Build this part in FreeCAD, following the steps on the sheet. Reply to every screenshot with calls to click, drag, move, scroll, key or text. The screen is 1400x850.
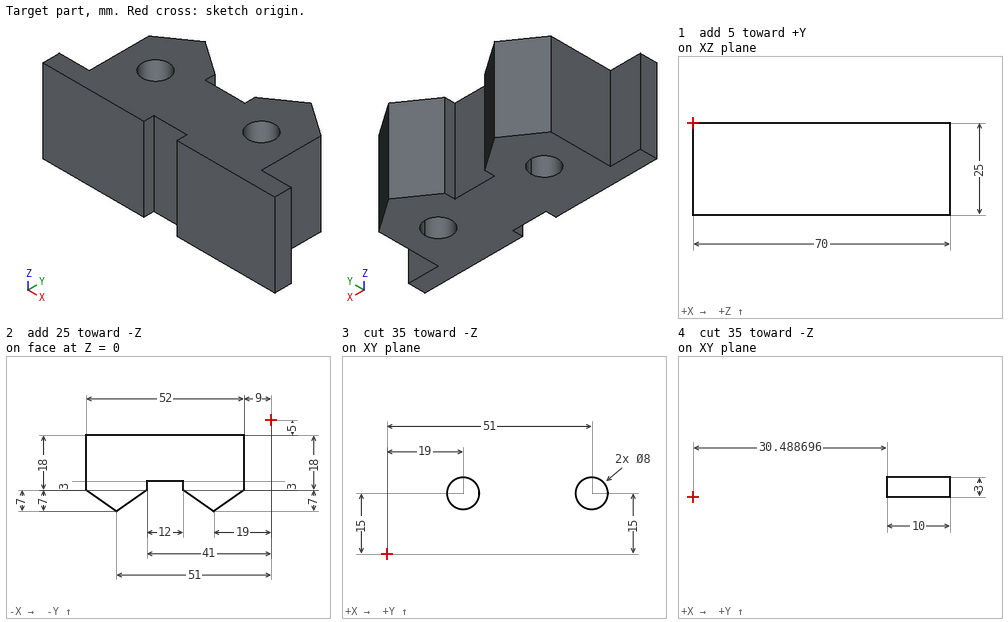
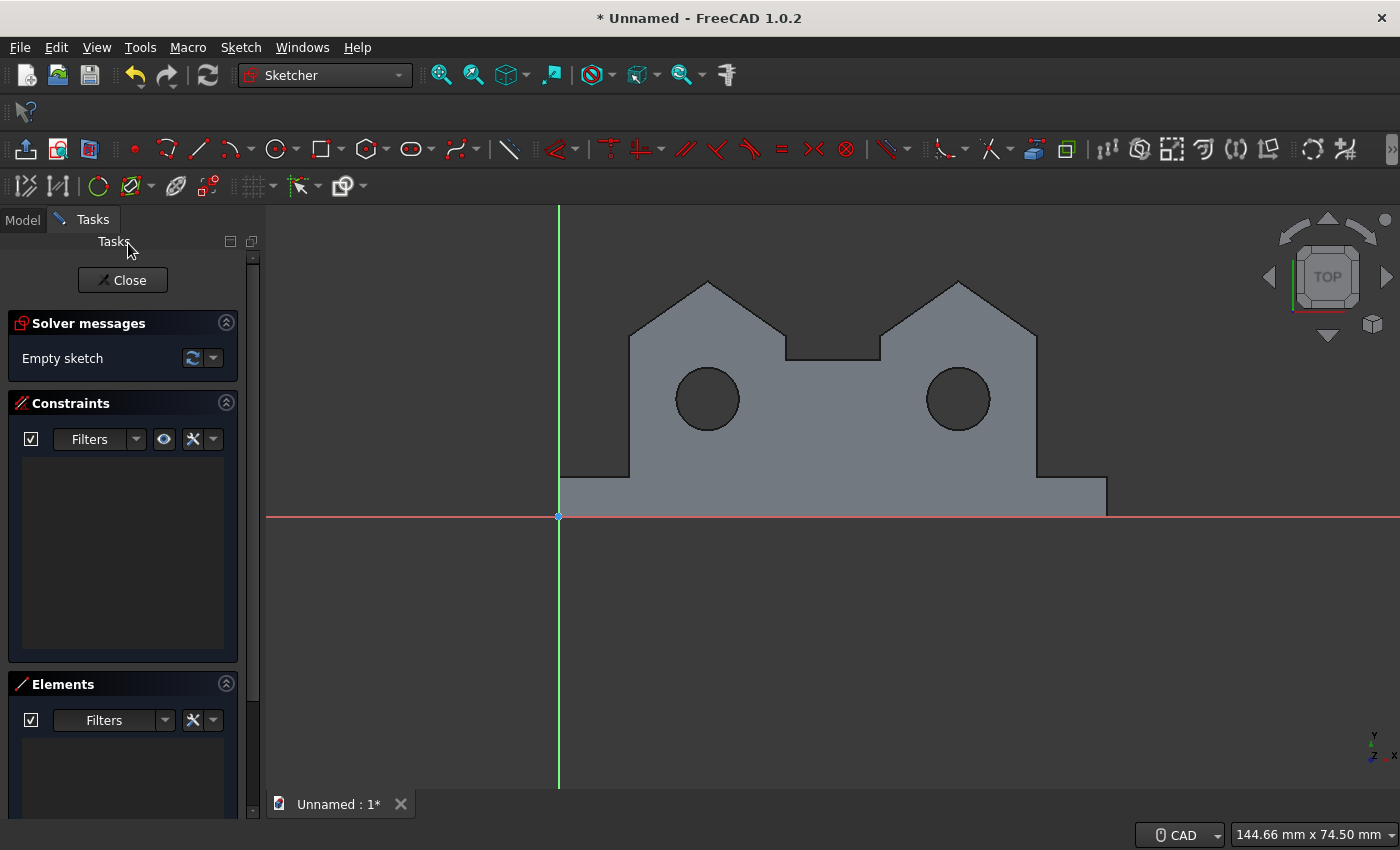
scroll(846, 506, up, 11)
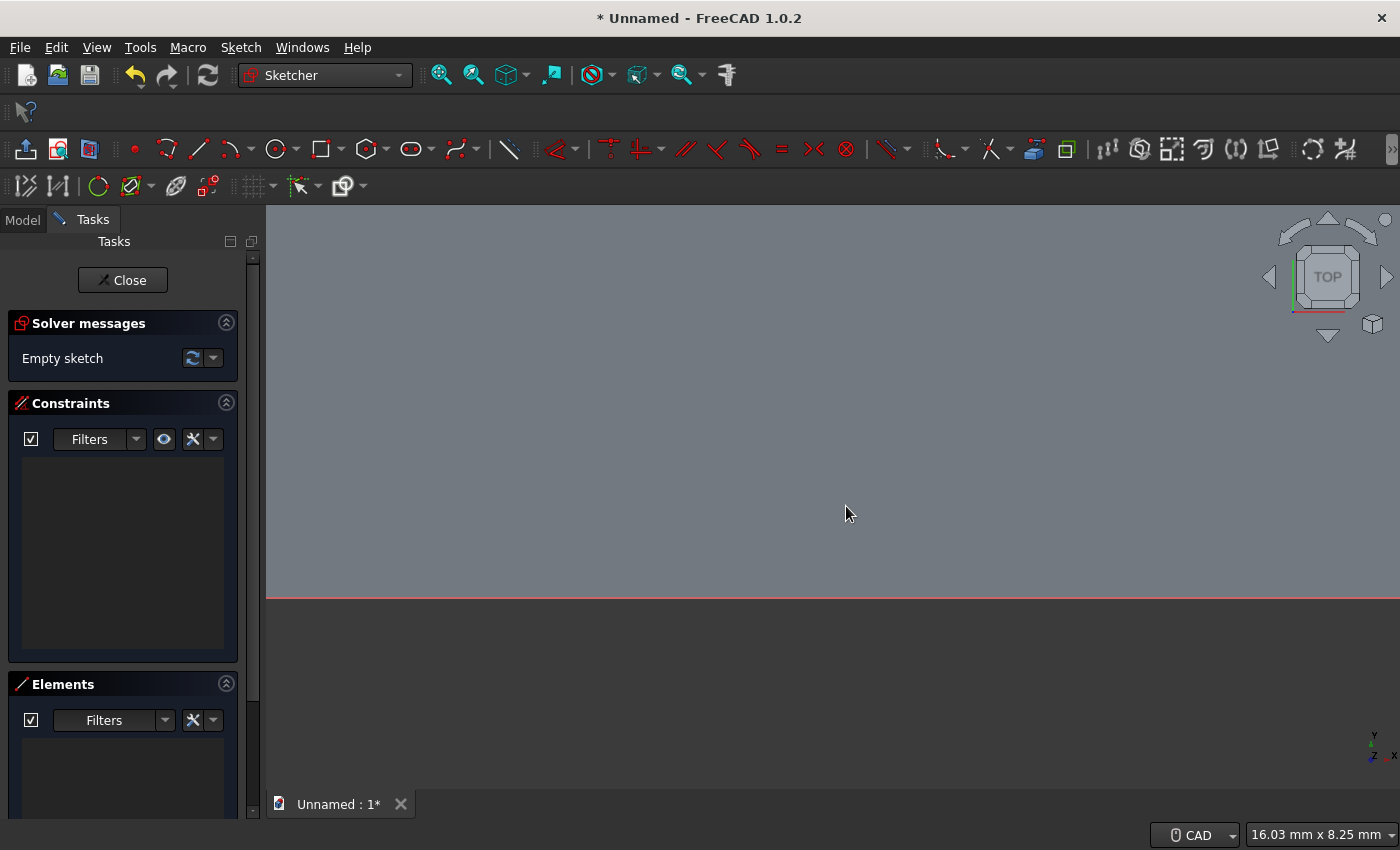
click(322, 150)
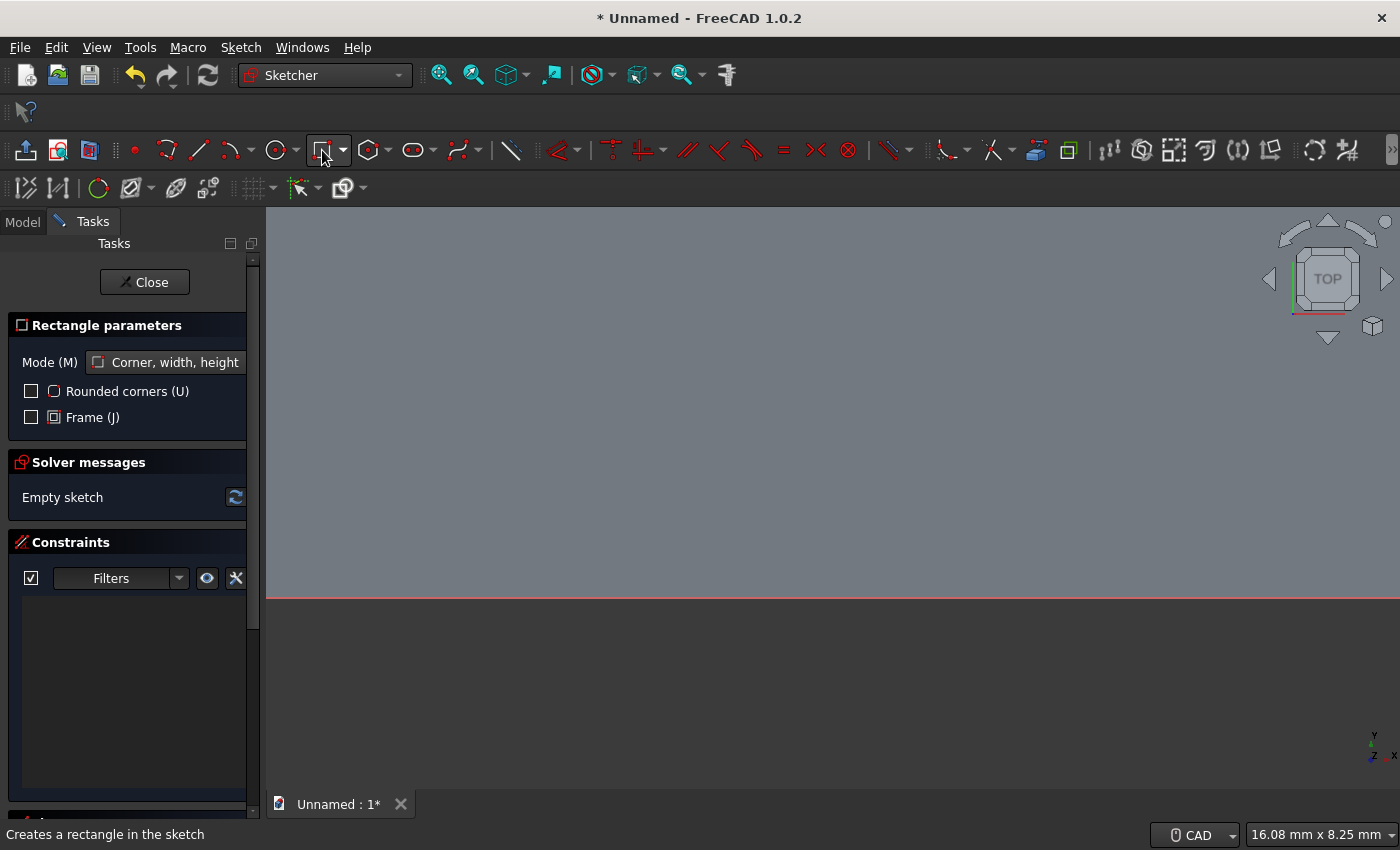
click(407, 387)
click(1112, 598)
key(Escape)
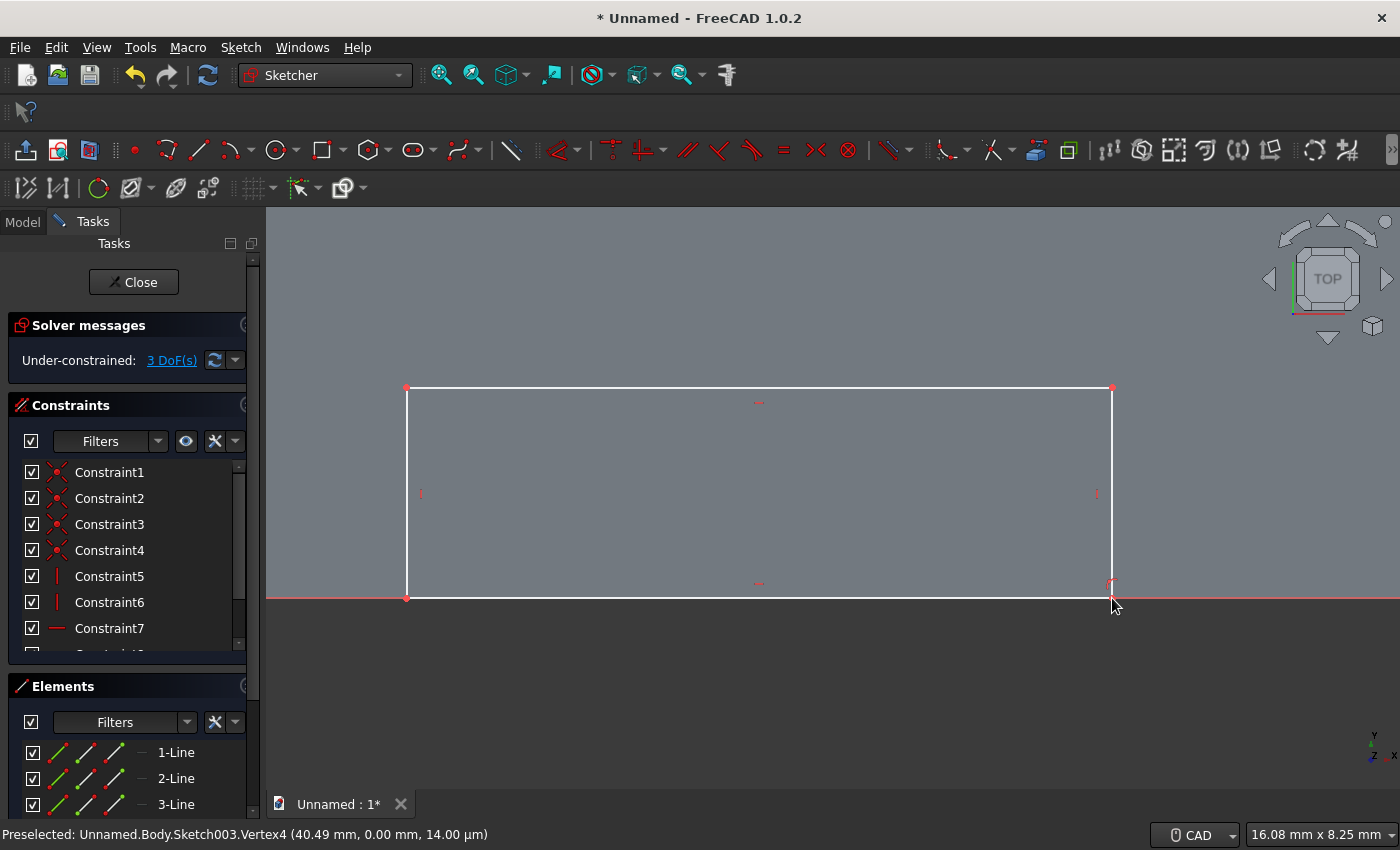
key(d)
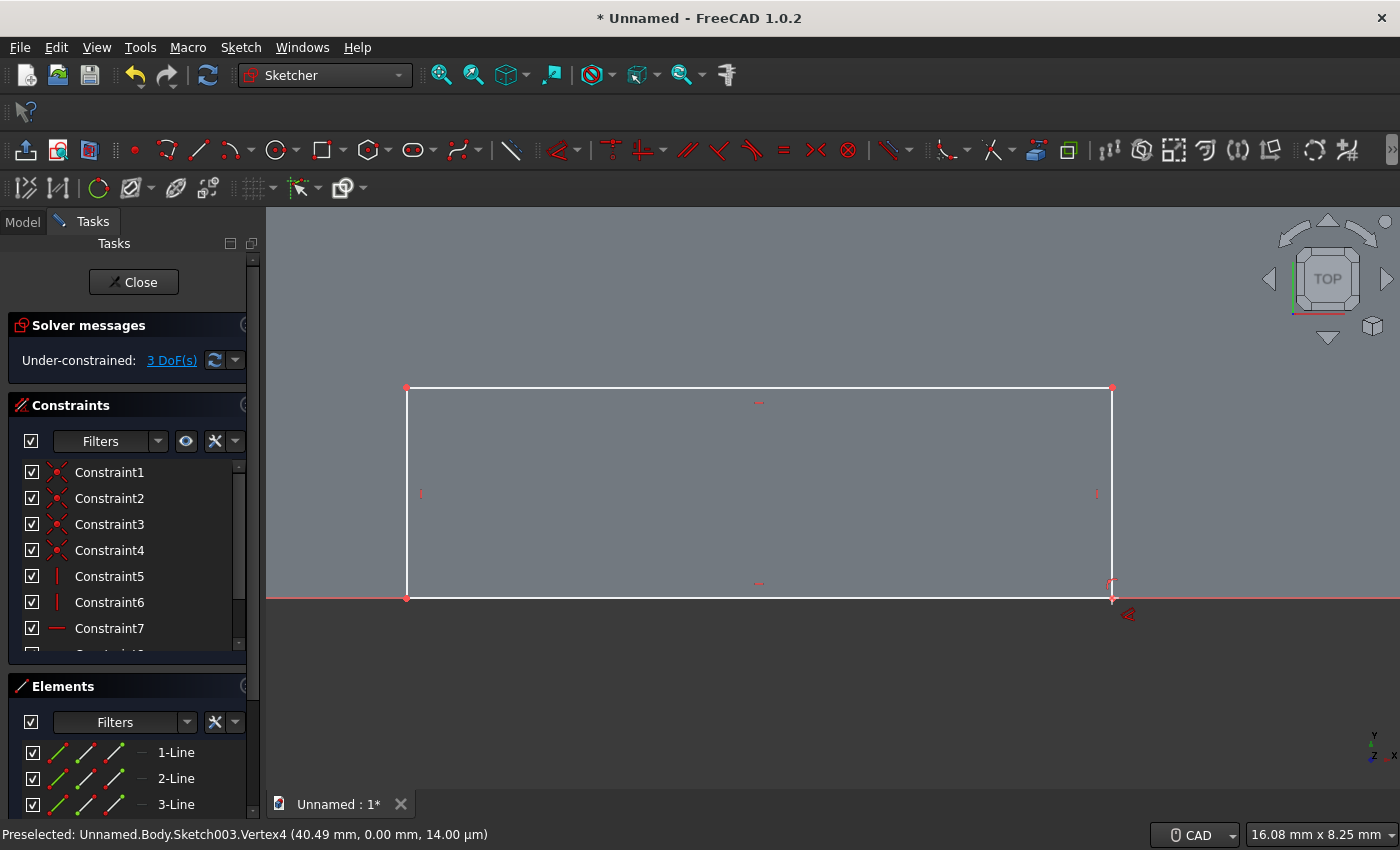
click(407, 451)
click(373, 493)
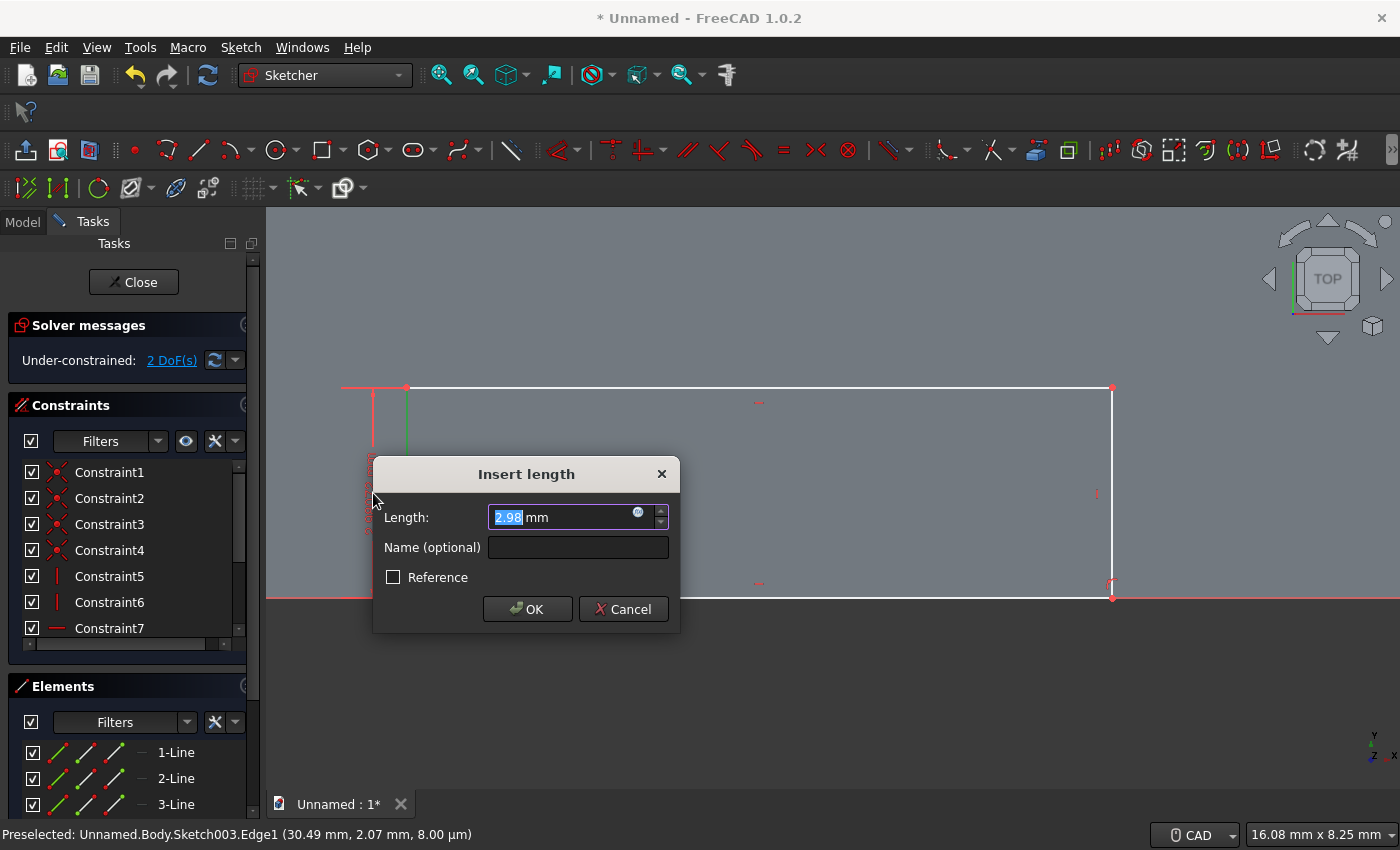
text(3)
key(Return)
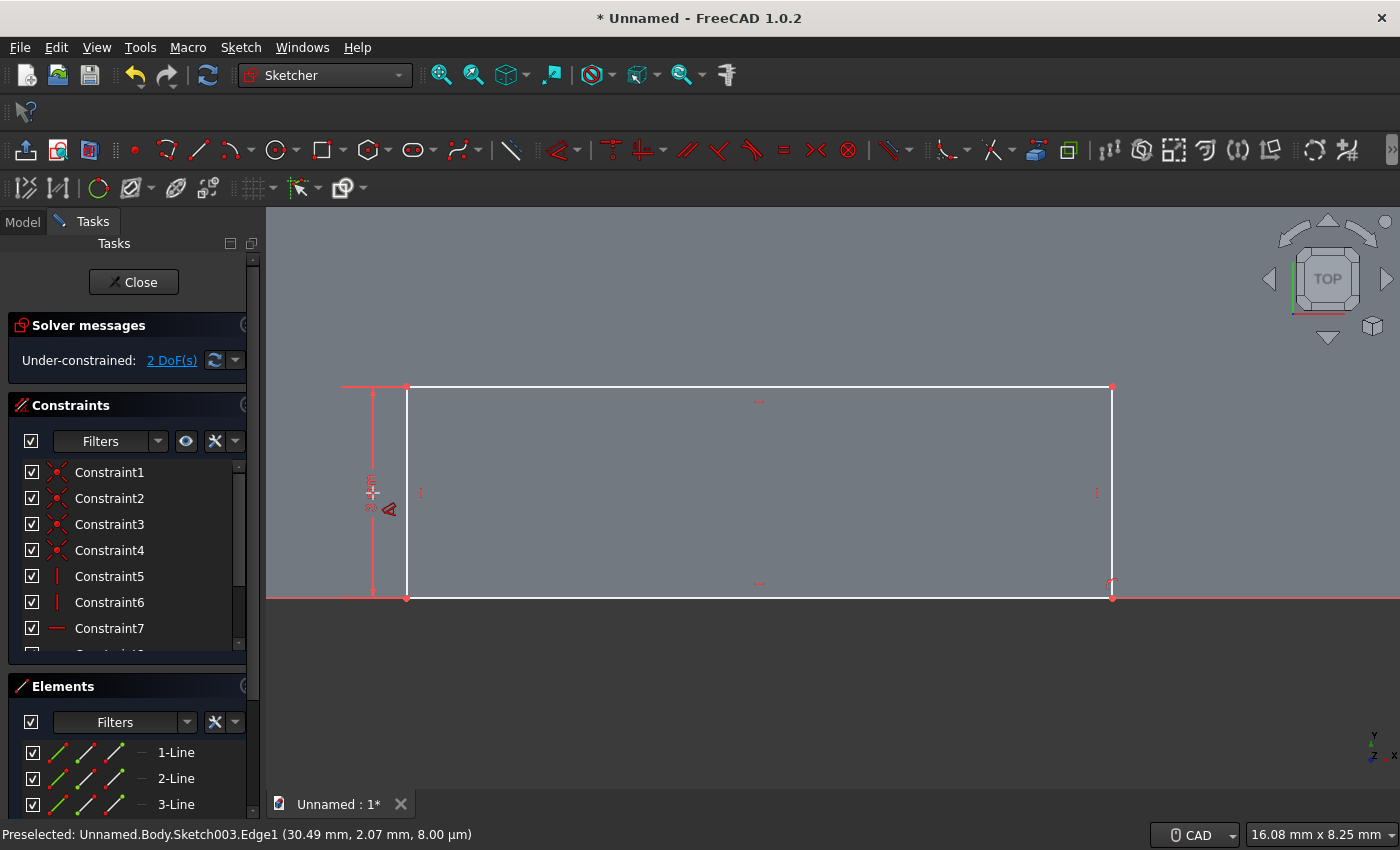
click(618, 598)
click(759, 632)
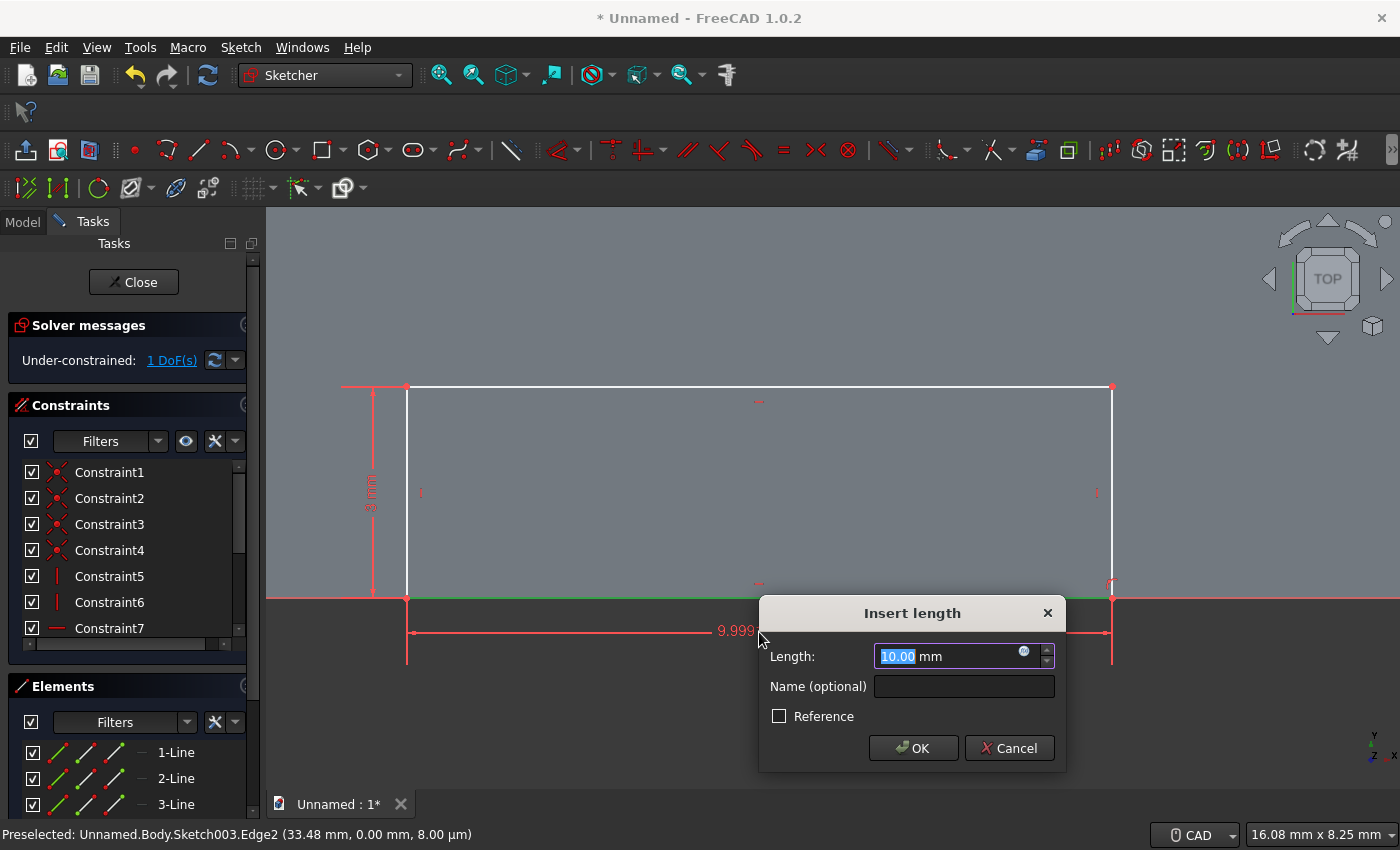
text(10)
key(Return)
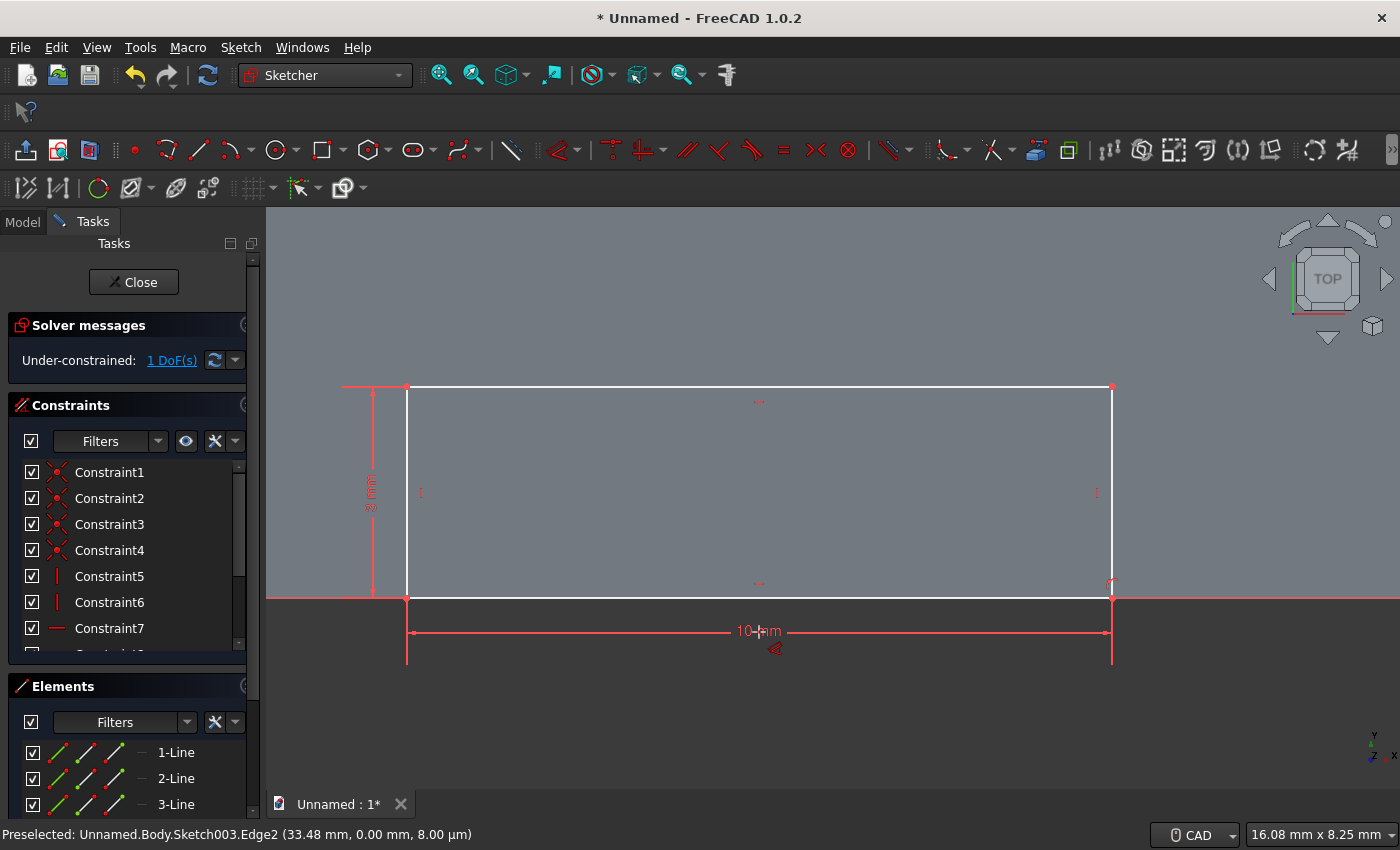
click(407, 387)
click(350, 632)